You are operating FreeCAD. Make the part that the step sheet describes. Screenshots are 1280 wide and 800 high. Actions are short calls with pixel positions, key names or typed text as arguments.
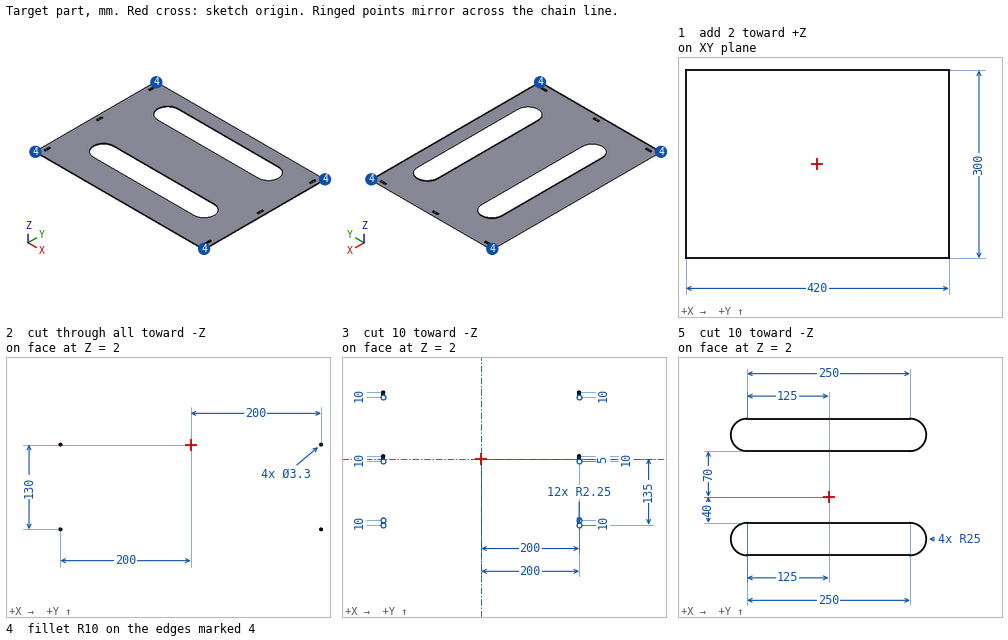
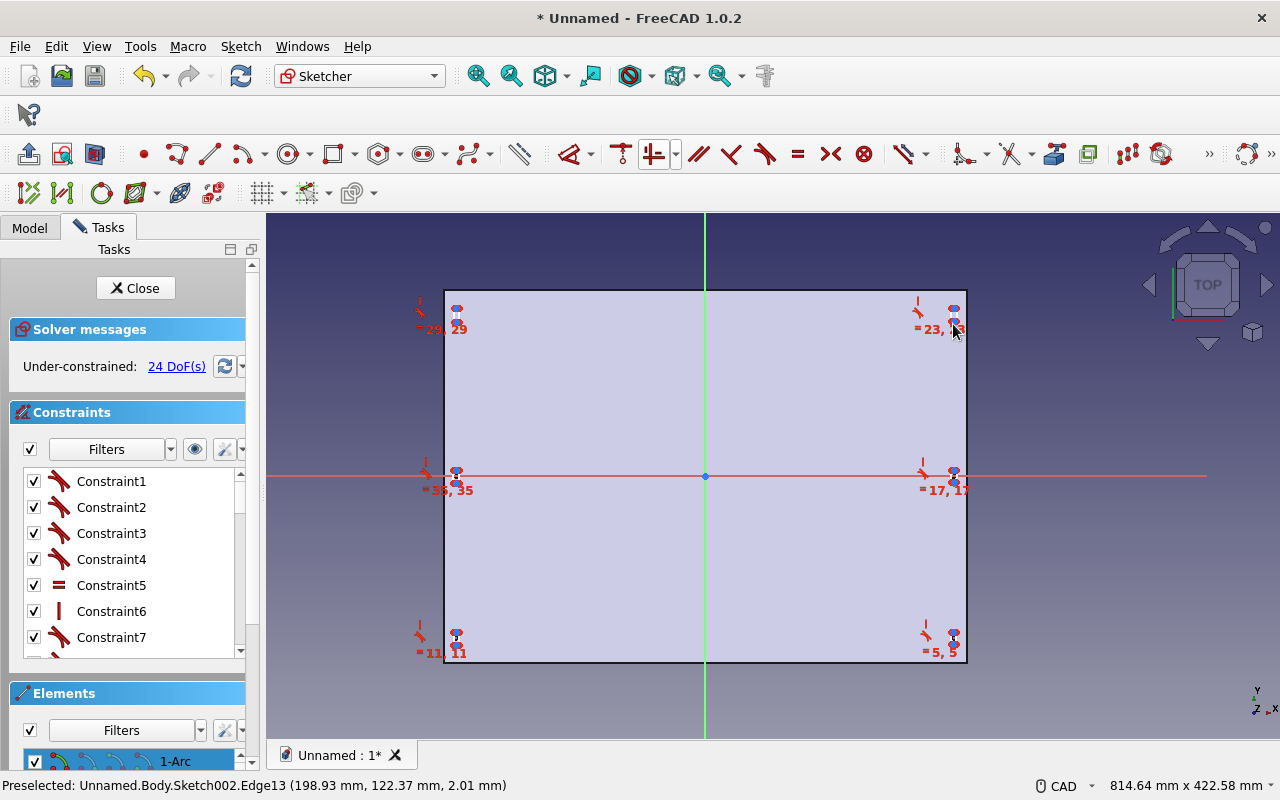
scroll(455, 324, up, 10)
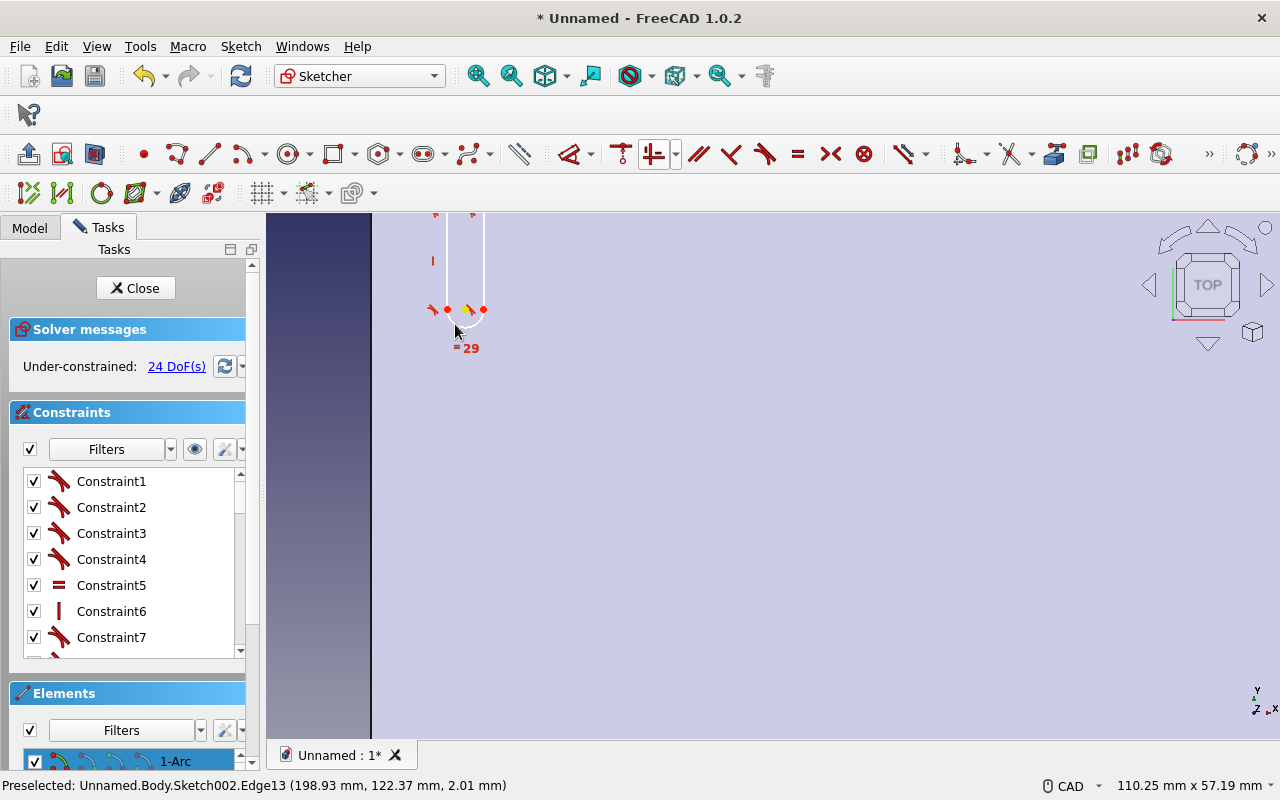
click(455, 324)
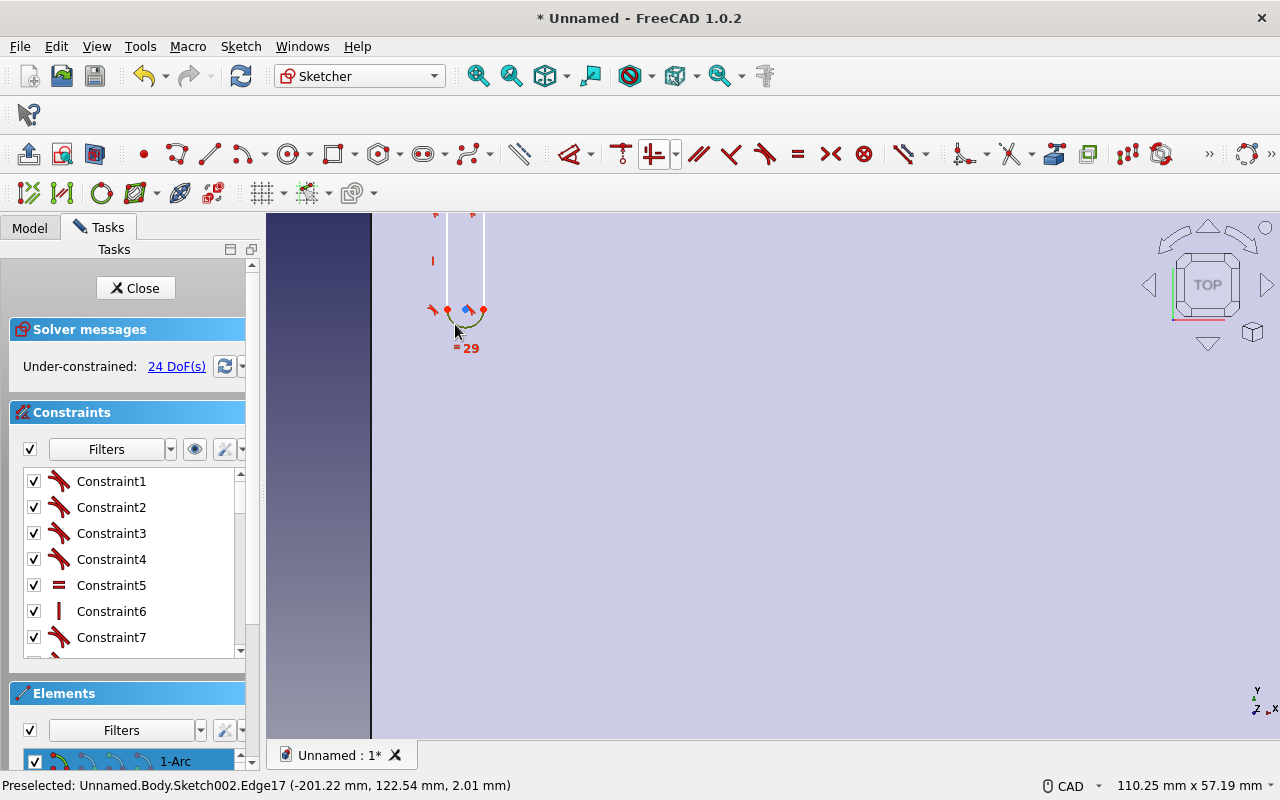
scroll(454, 324, down, 10)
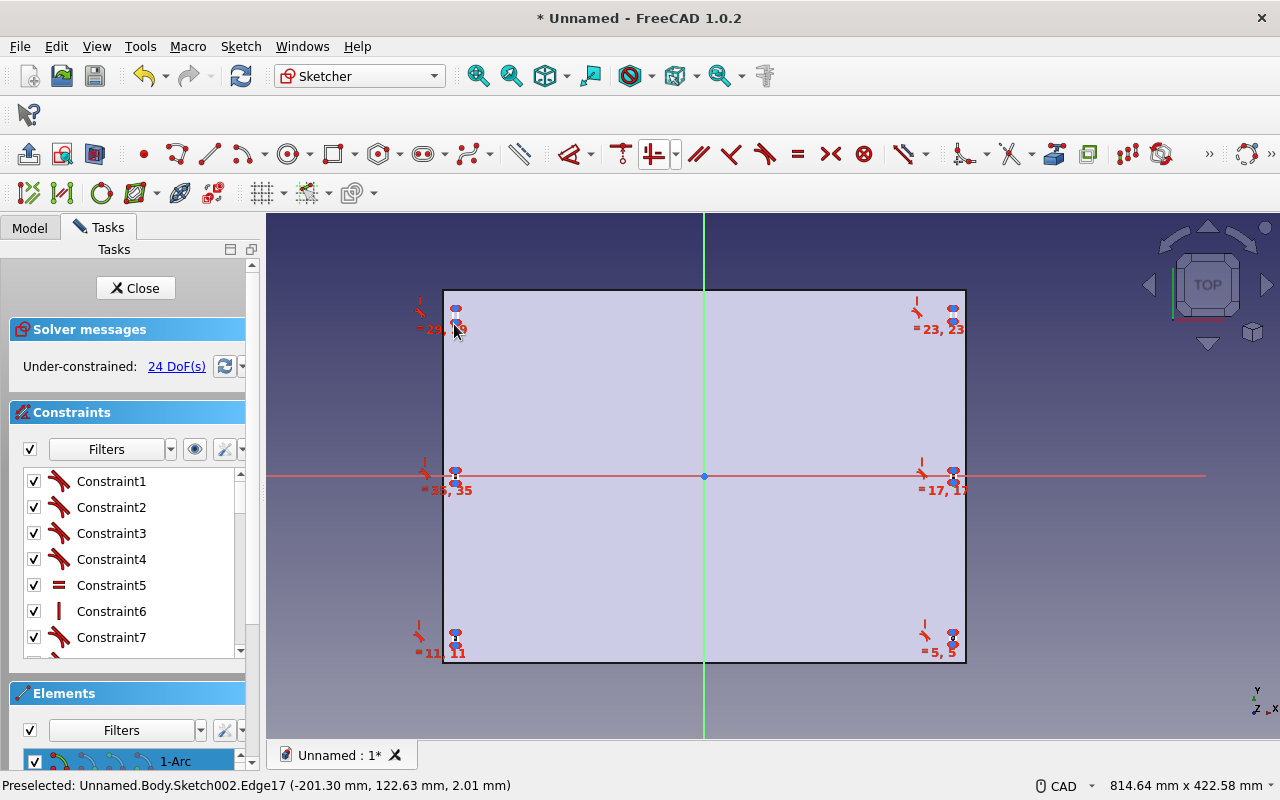
scroll(454, 485, up, 9)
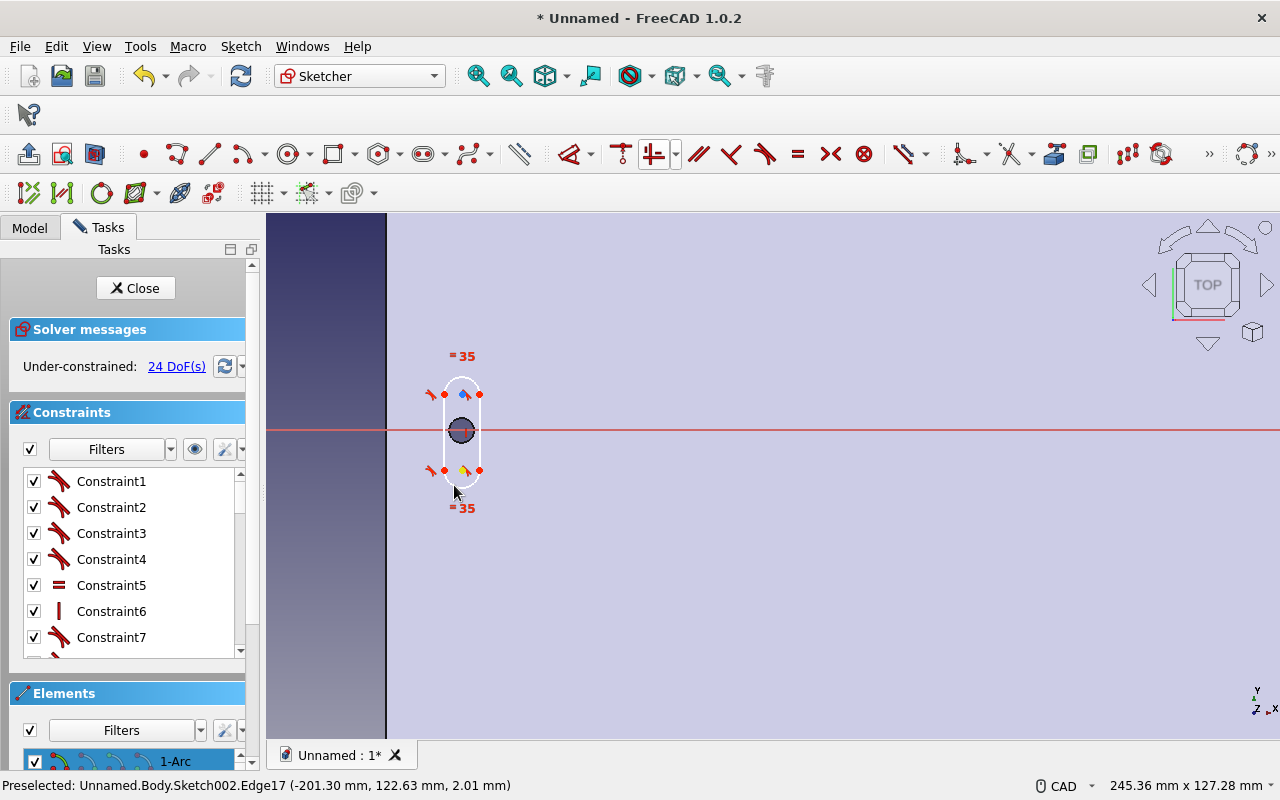
click(452, 485)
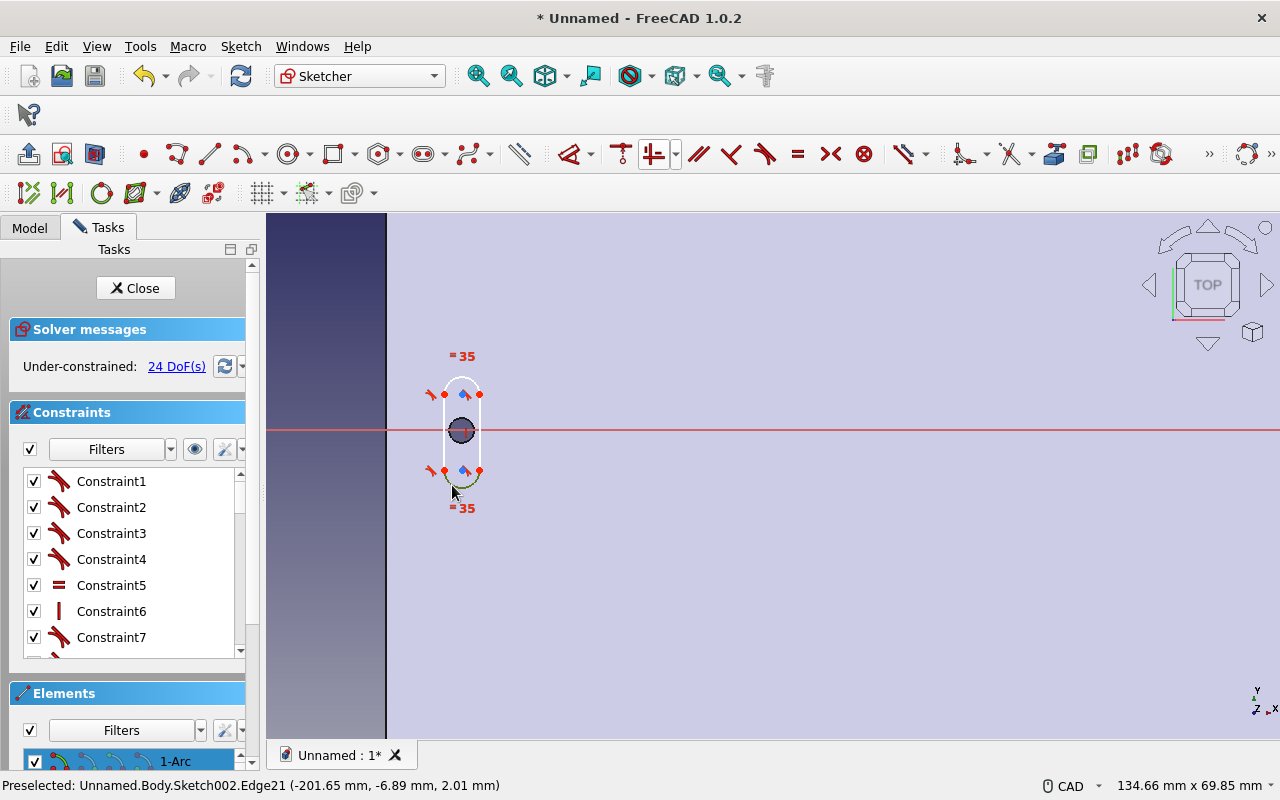
key(e)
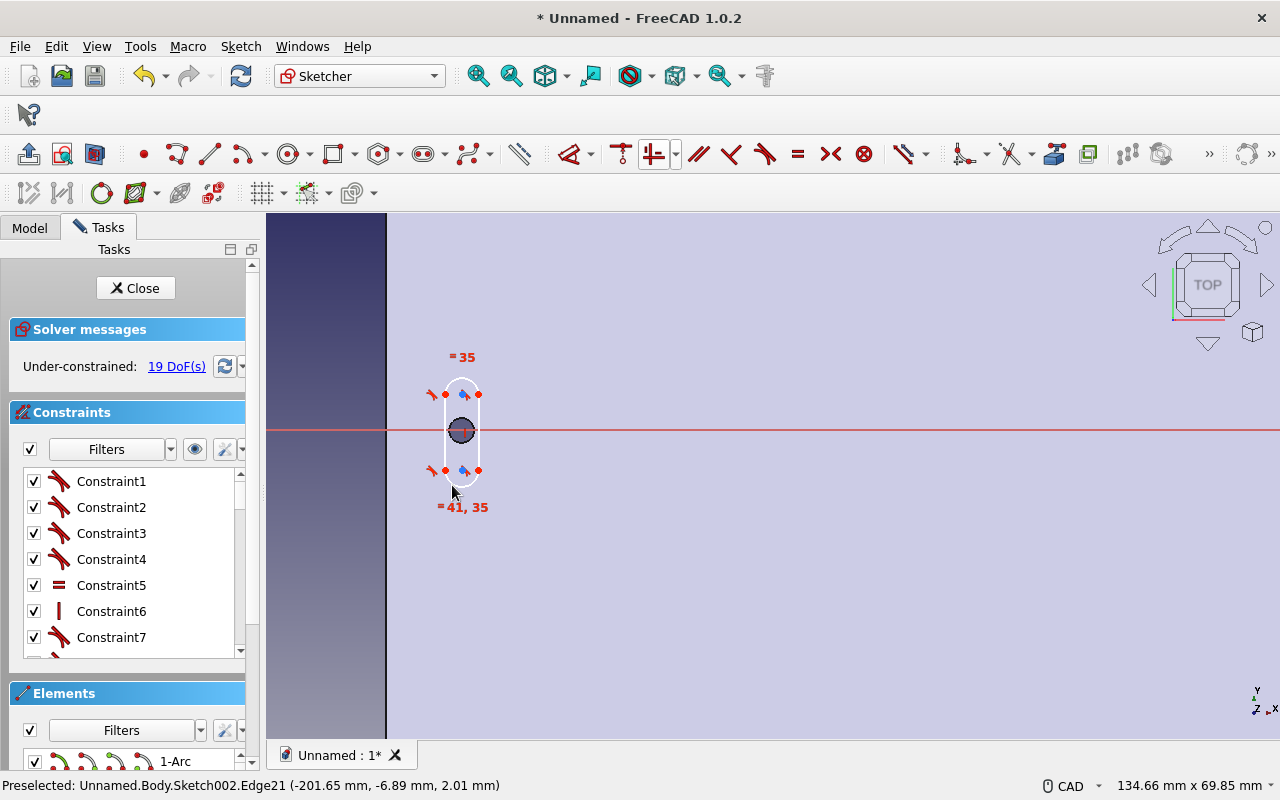
scroll(454, 485, down, 9)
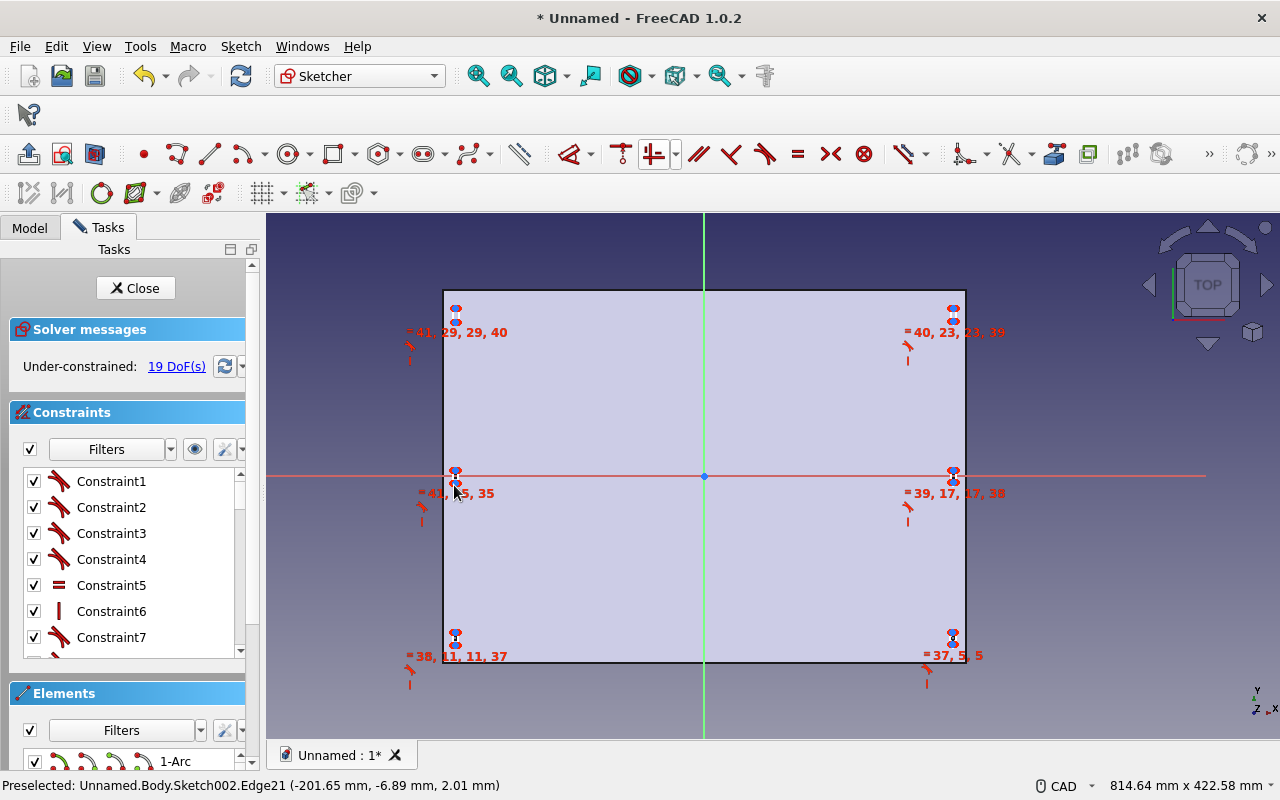
scroll(953, 645, up, 8)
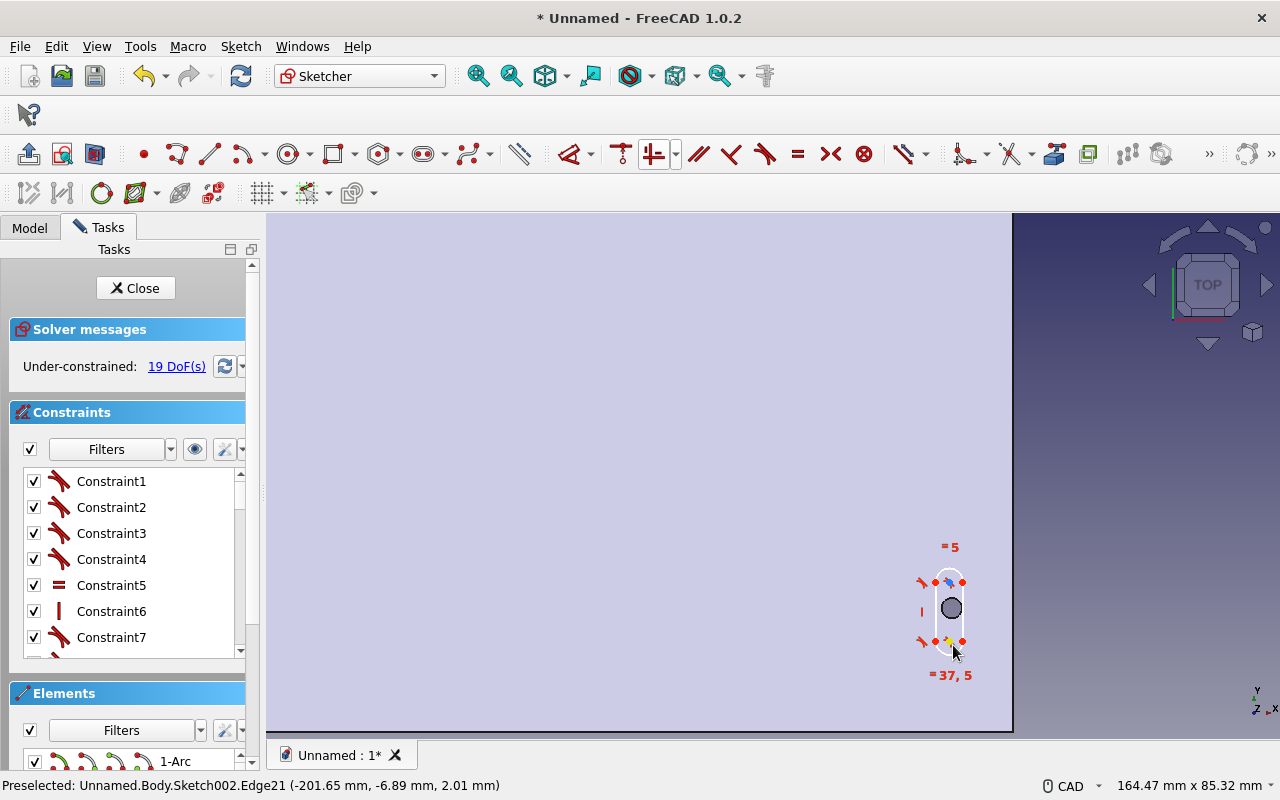
click(949, 641)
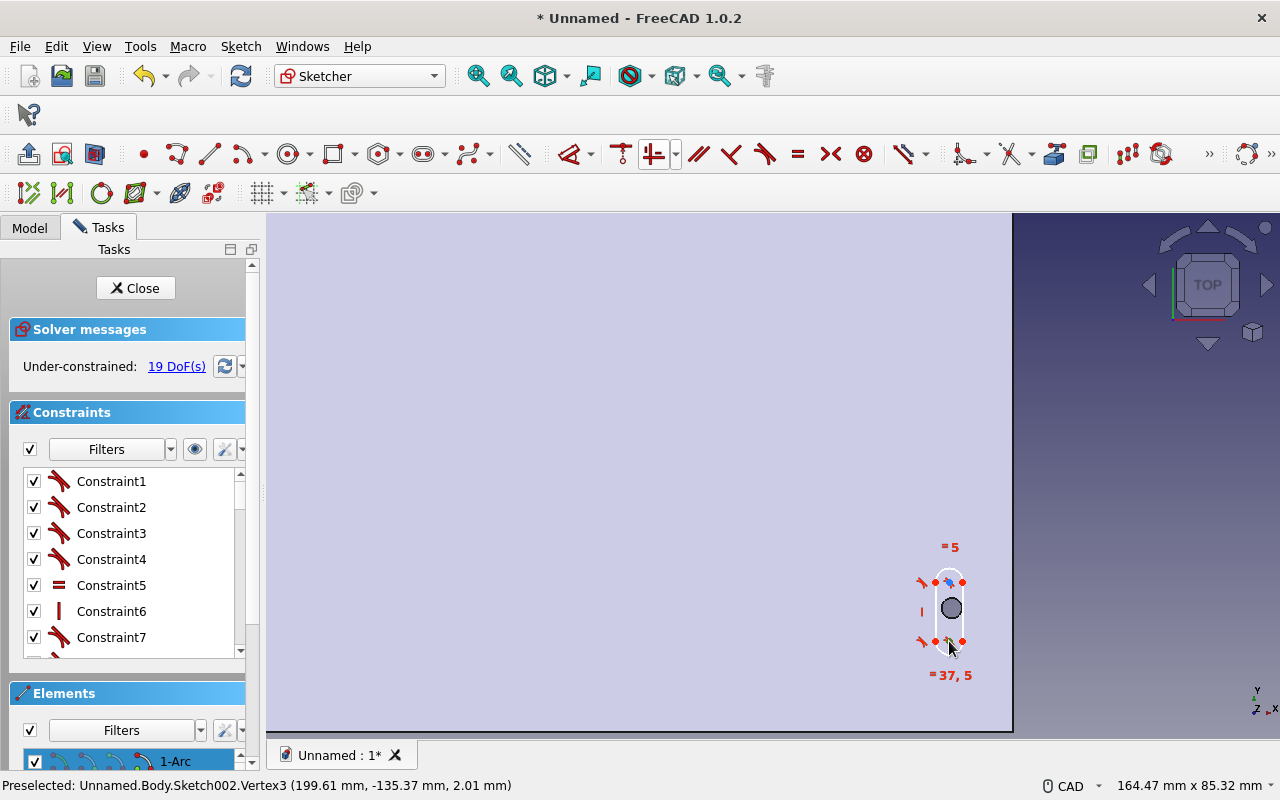
scroll(954, 645, down, 8)